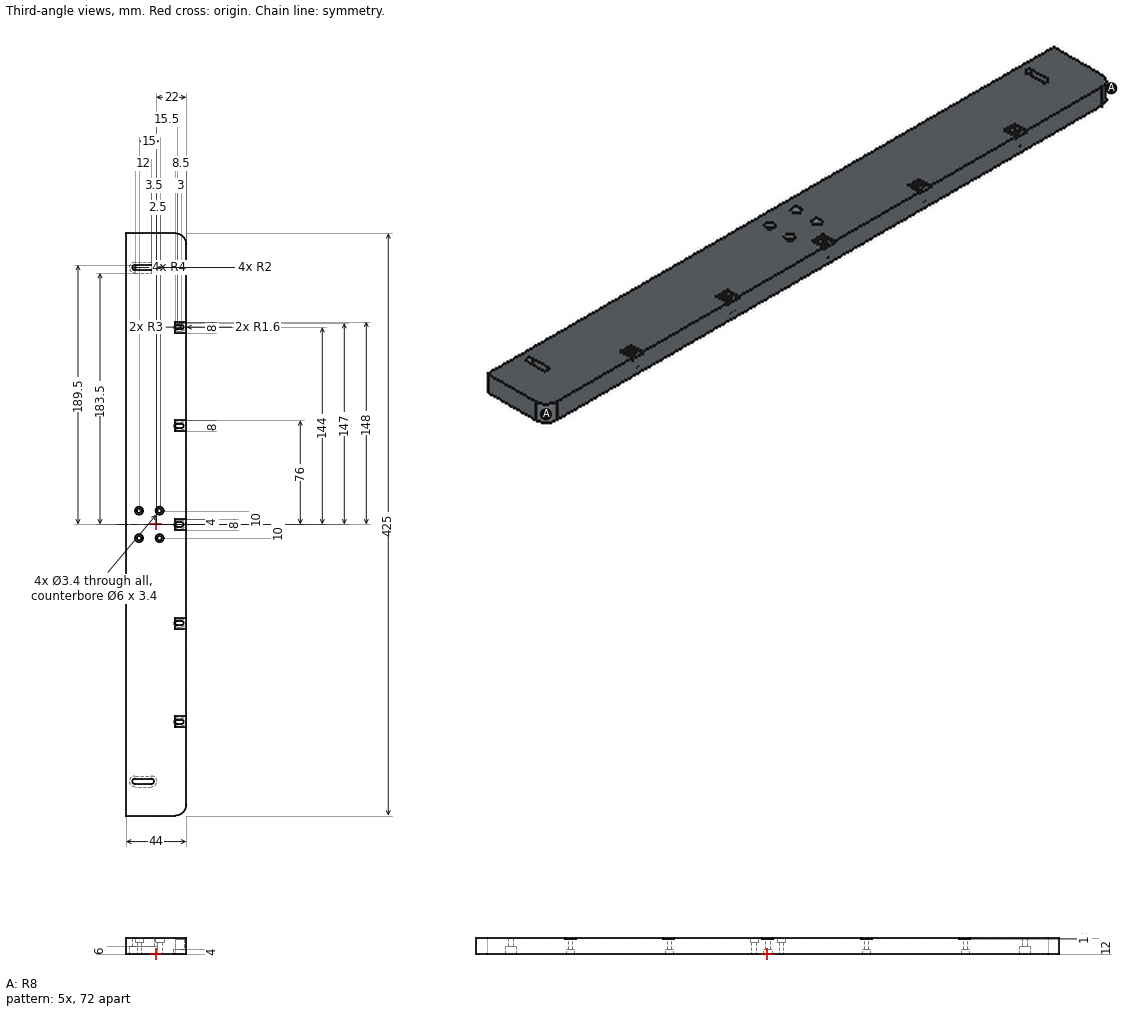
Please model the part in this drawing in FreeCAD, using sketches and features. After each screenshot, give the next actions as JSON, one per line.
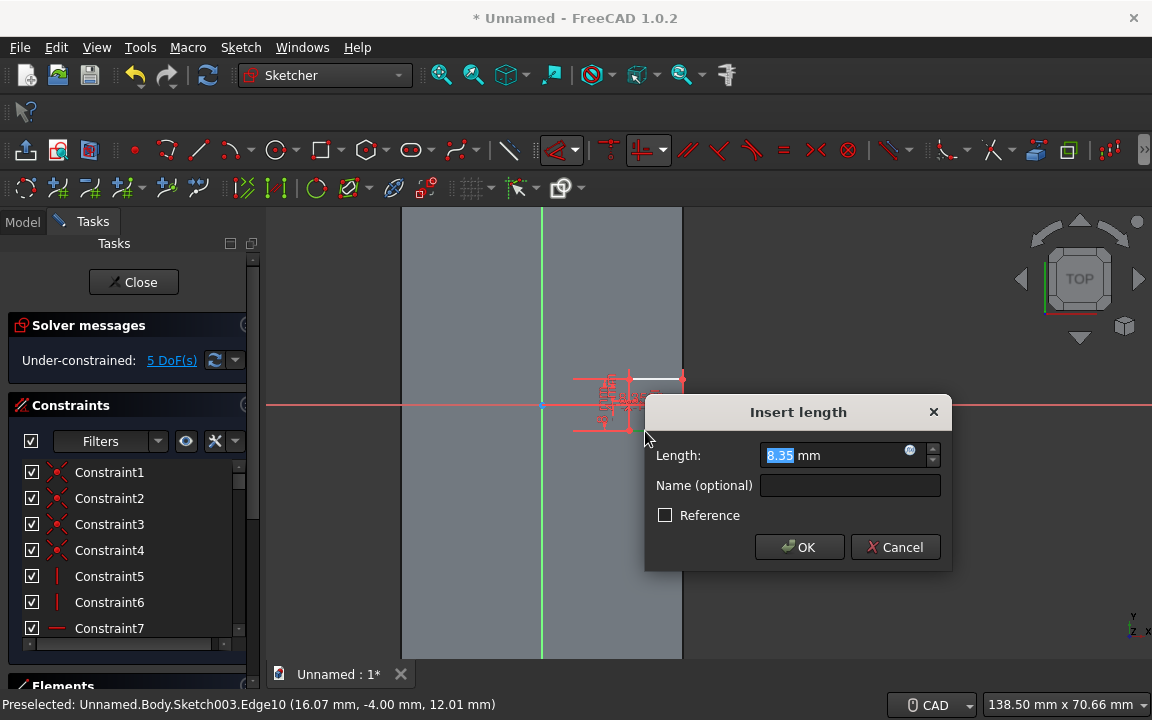
{"action": "type", "text": "8.5"}
{"action": "key", "text": "Return"}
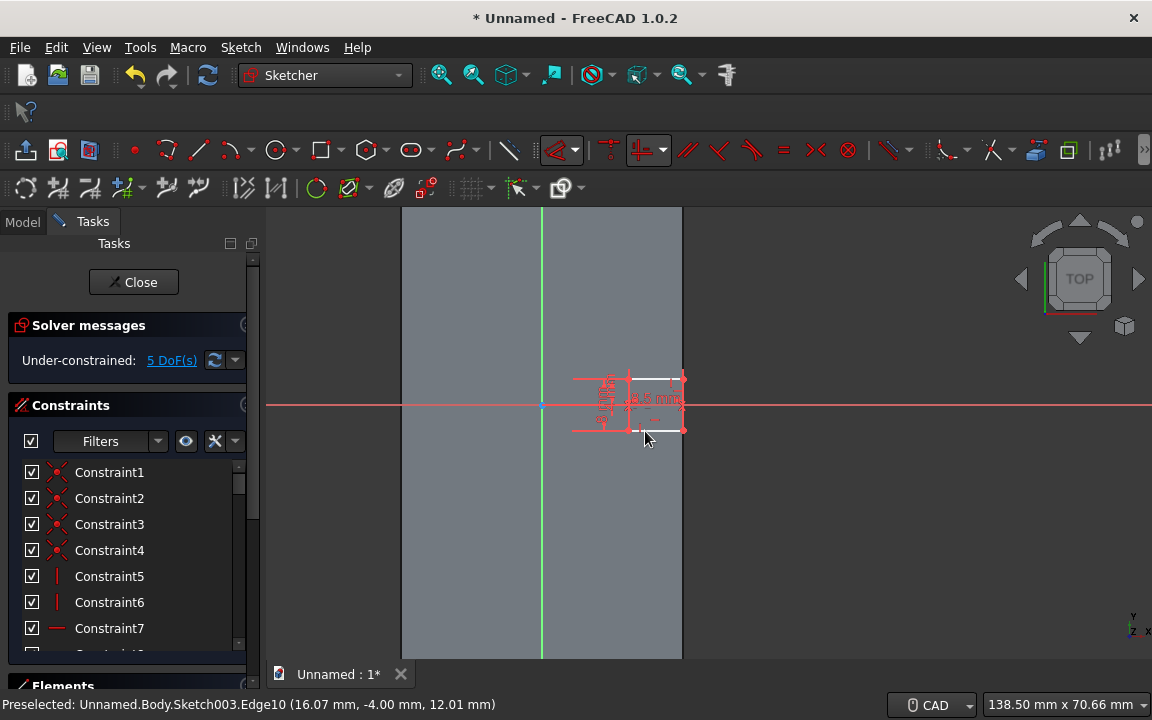
{"action": "scroll", "coordinate": [645, 437], "scroll_direction": "down", "scroll_amount": 10}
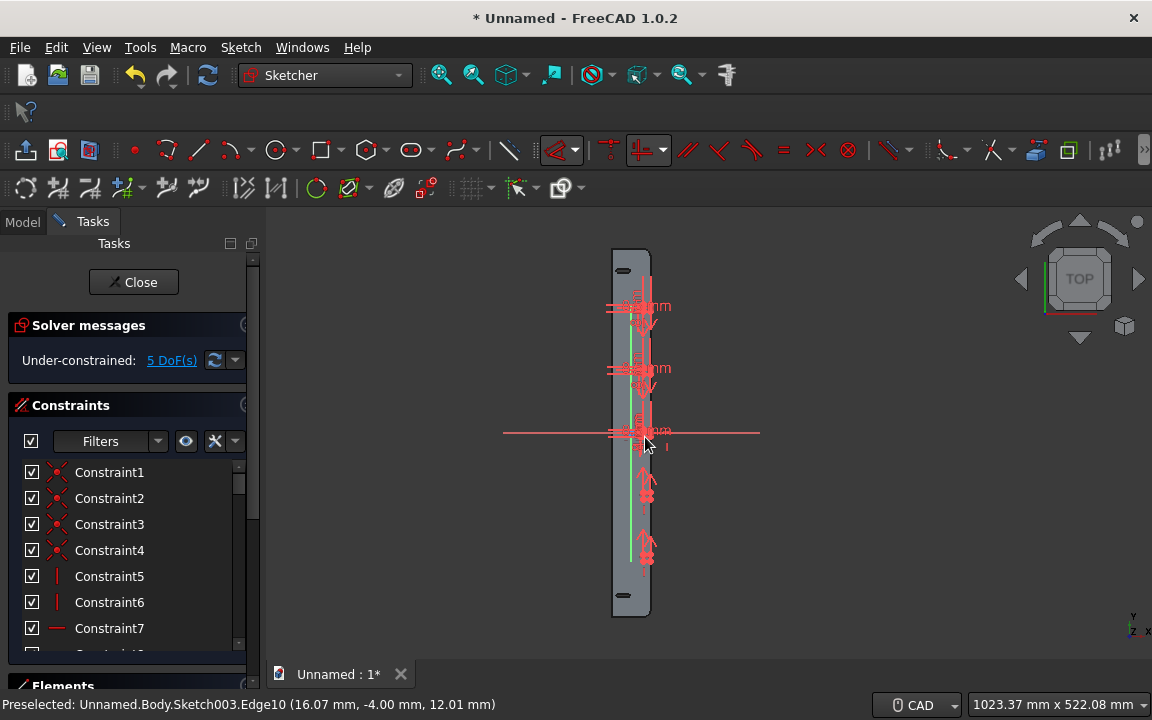
{"action": "scroll", "coordinate": [651, 312], "scroll_direction": "up", "scroll_amount": 4}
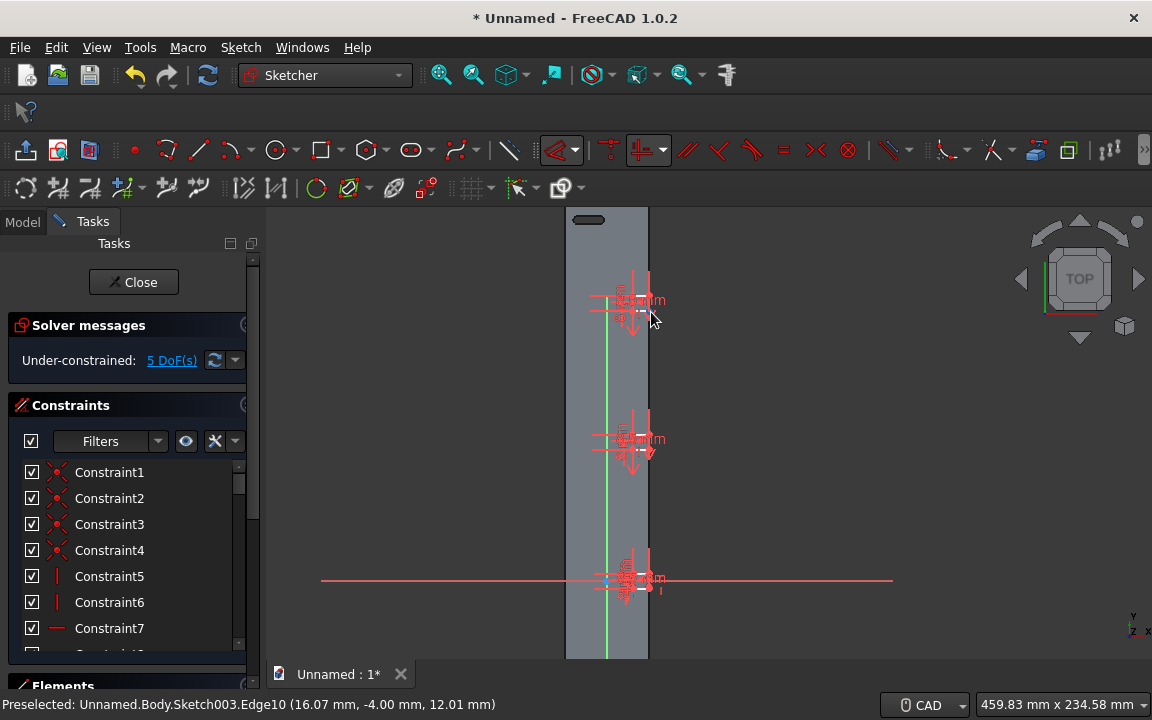
{"action": "left_click", "coordinate": [649, 311]}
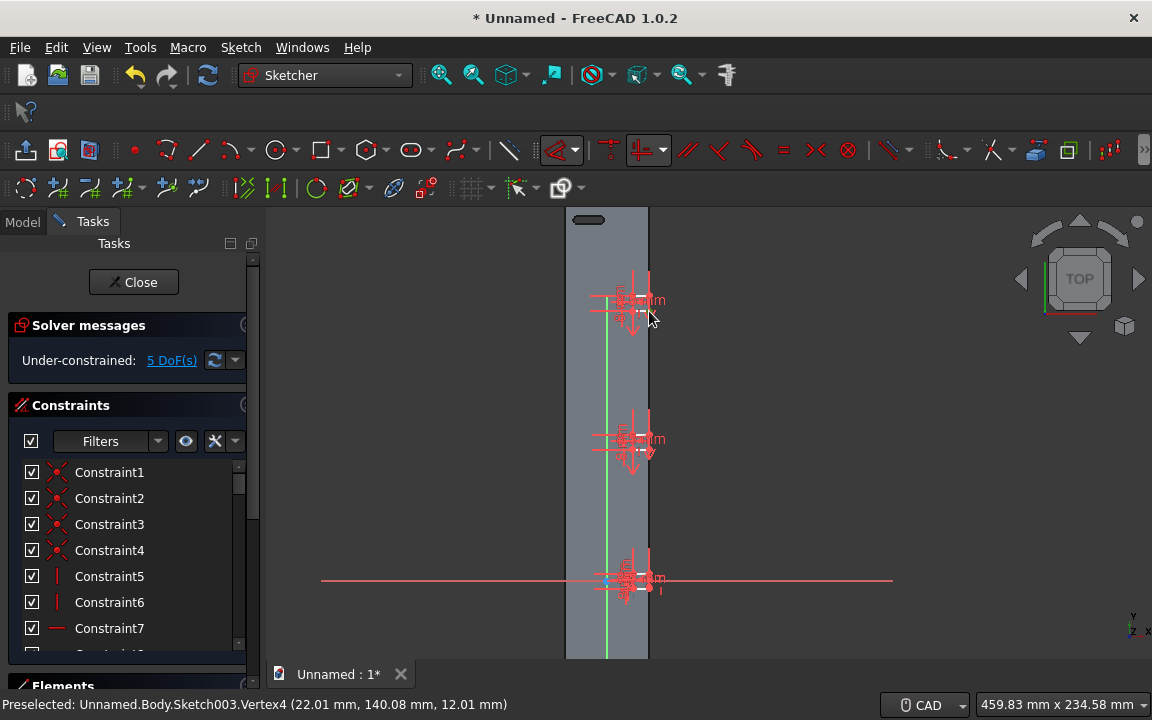
{"action": "key", "text": "l"}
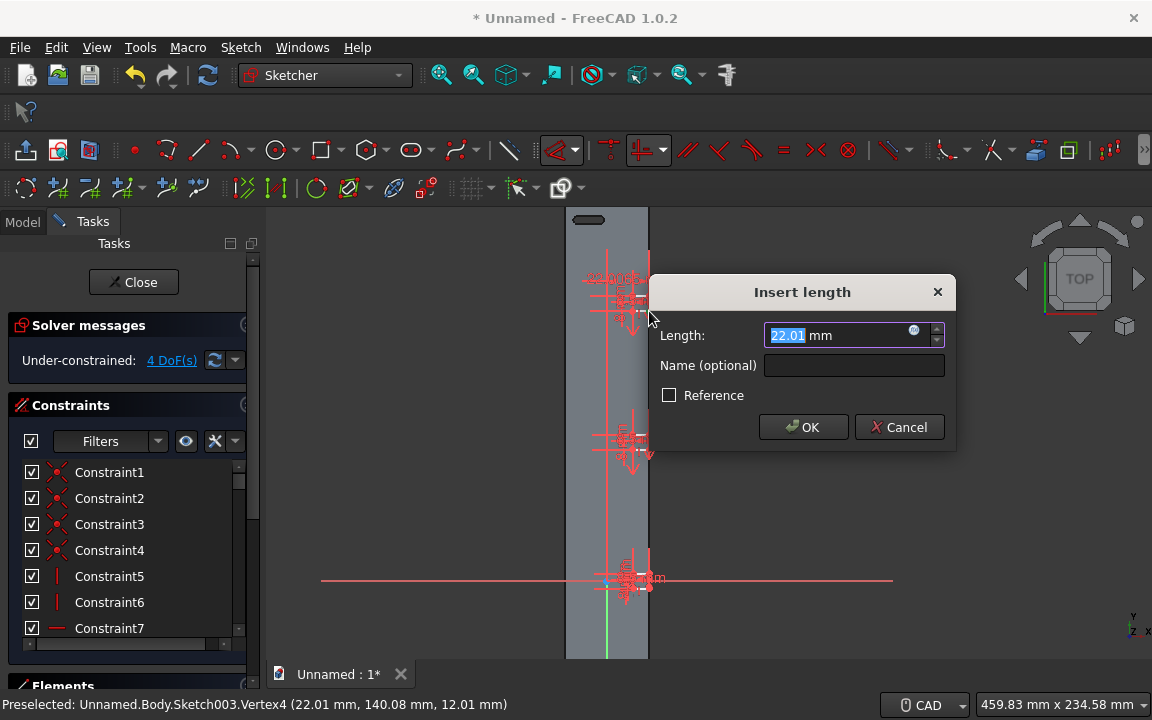
{"action": "type", "text": "22"}
{"action": "key", "text": "Return"}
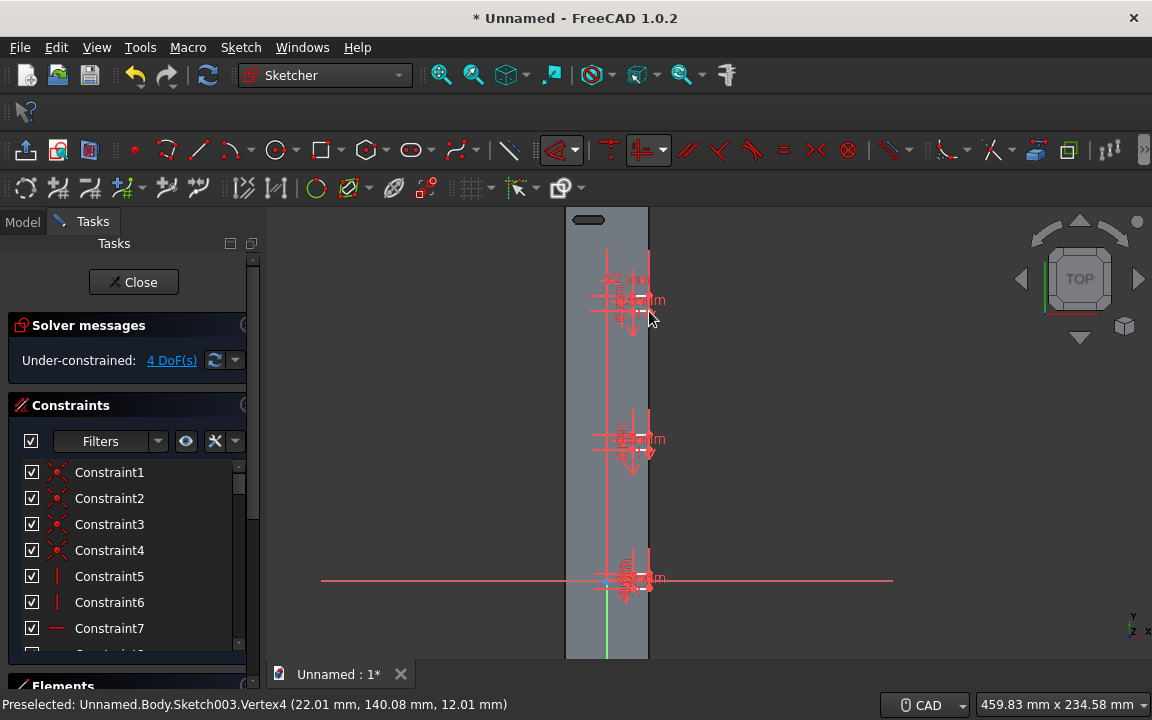
{"action": "left_click", "coordinate": [633, 435]}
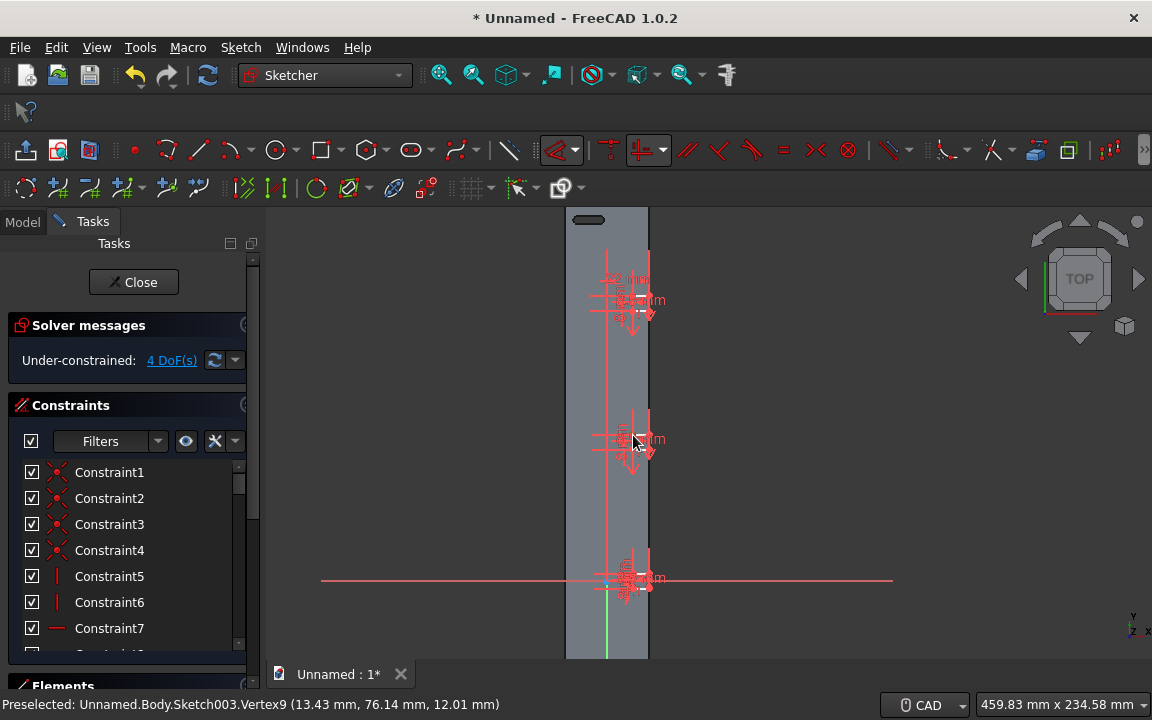
{"action": "key", "text": "i"}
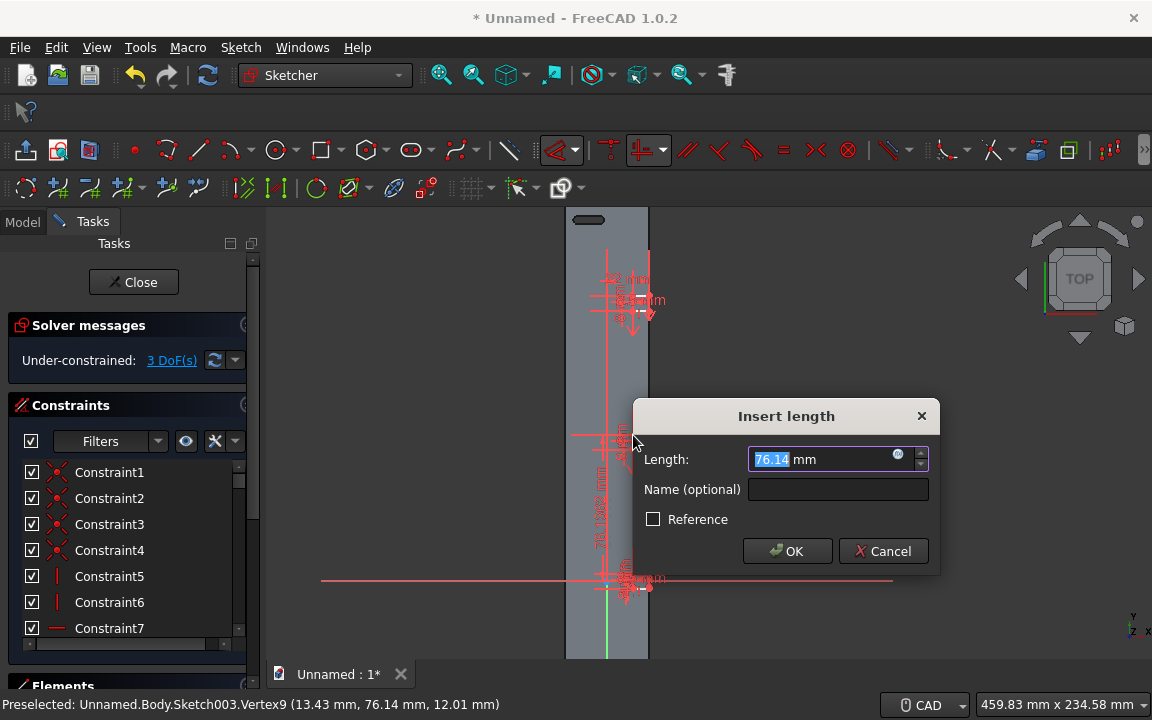
{"action": "type", "text": "76"}
{"action": "key", "text": "Return"}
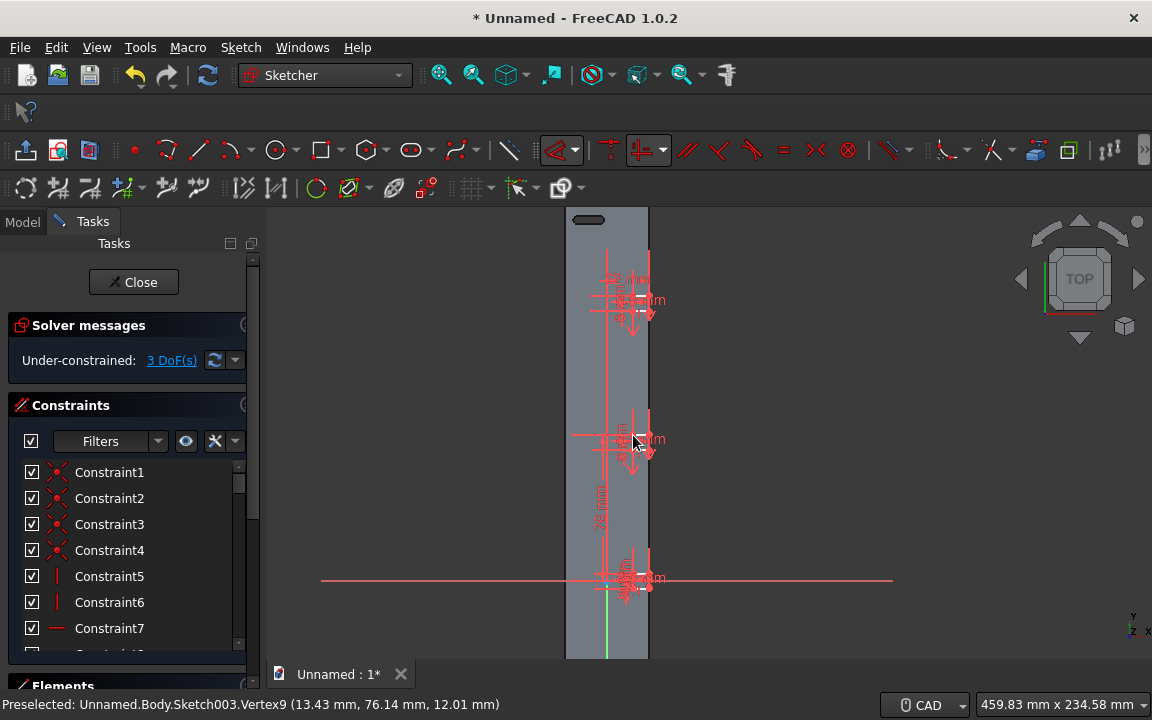
{"action": "left_click", "coordinate": [649, 450]}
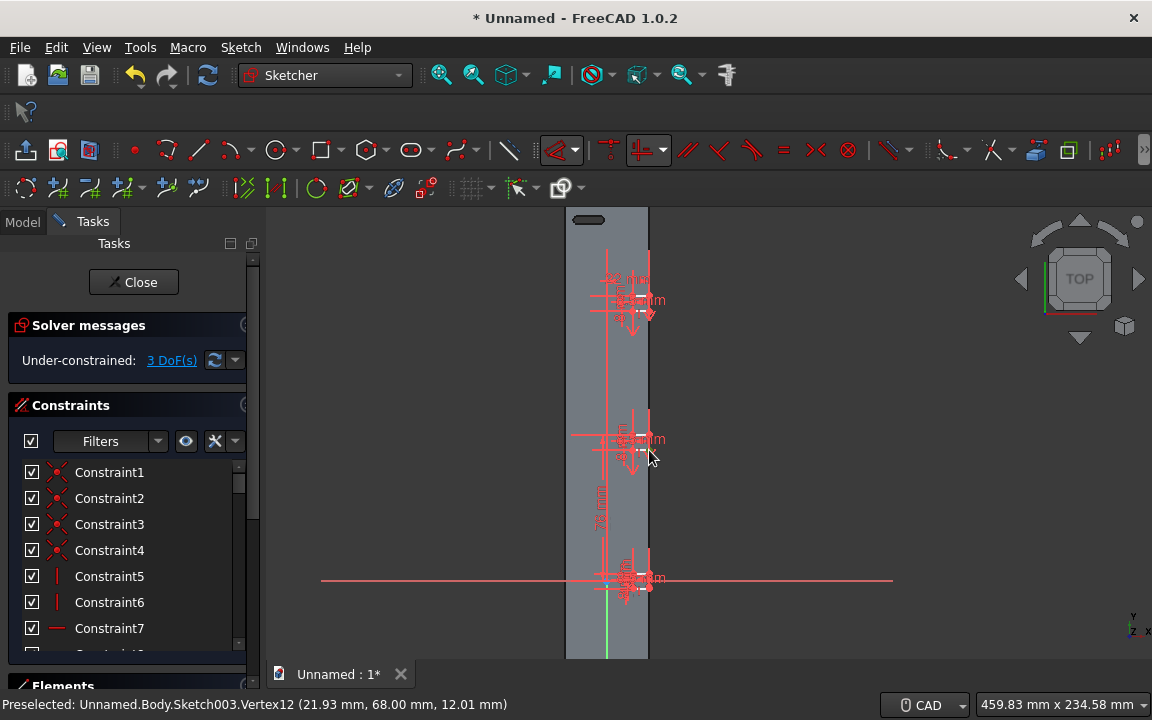
{"action": "key", "text": "l"}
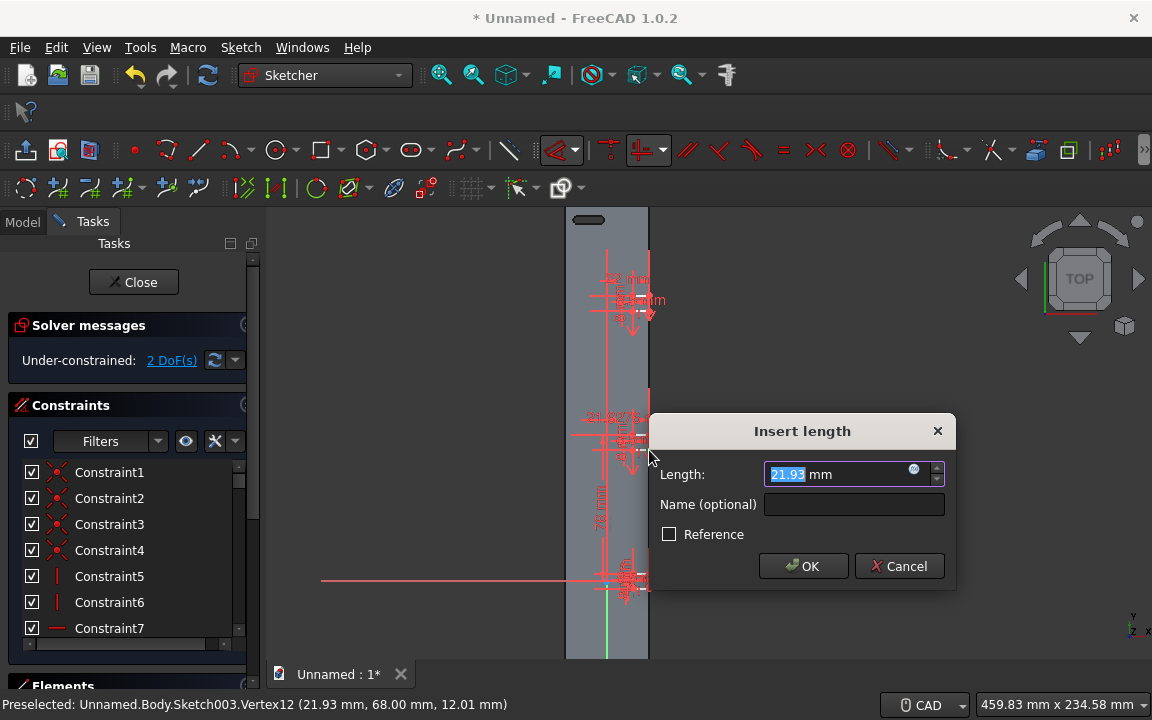
{"action": "type", "text": "22"}
{"action": "key", "text": "Return"}